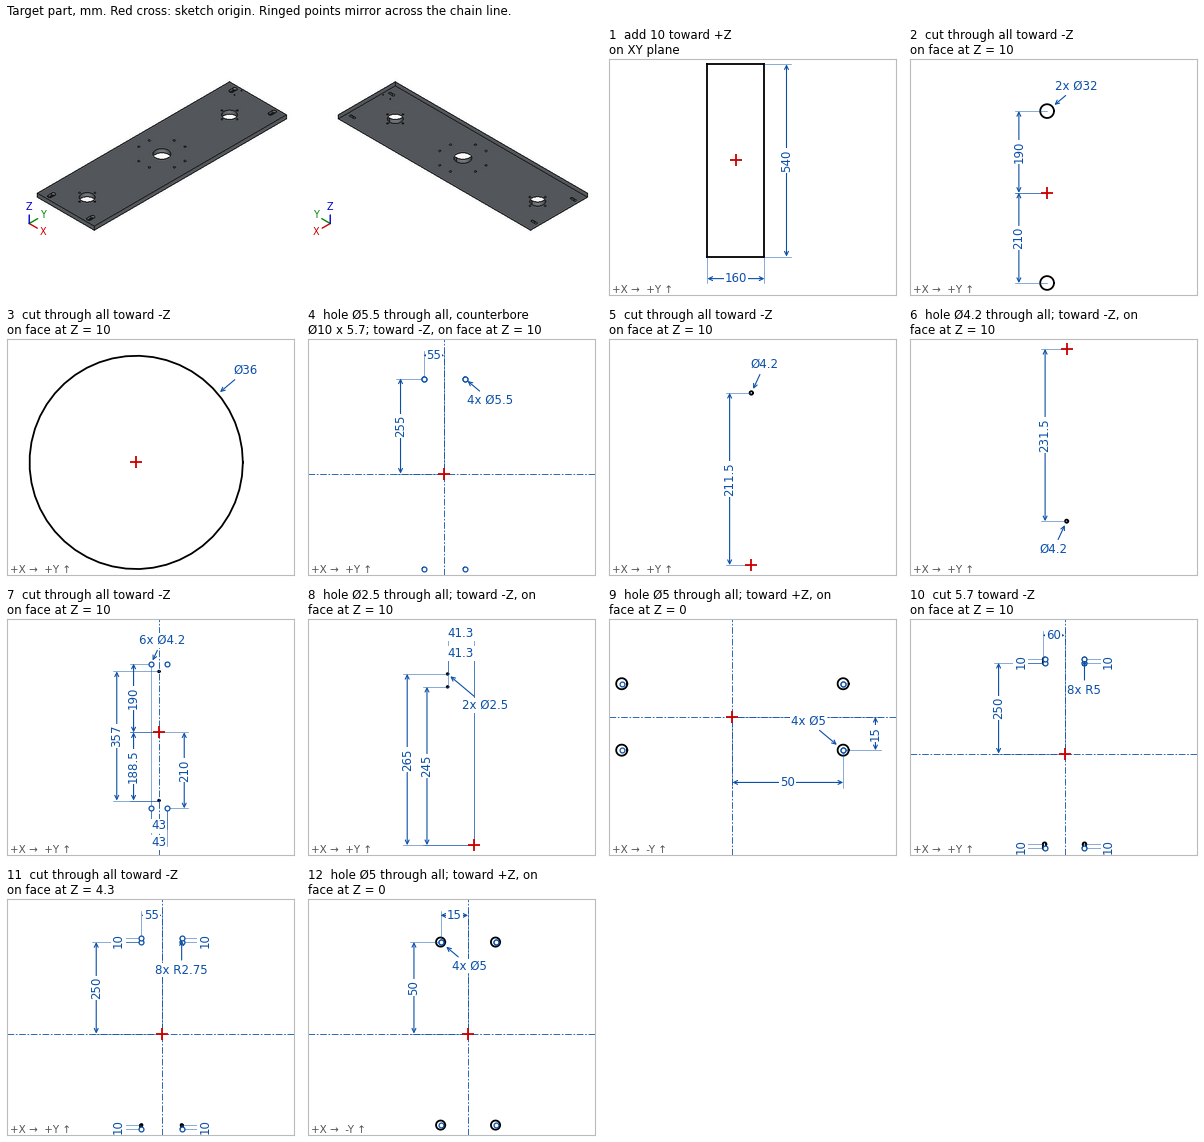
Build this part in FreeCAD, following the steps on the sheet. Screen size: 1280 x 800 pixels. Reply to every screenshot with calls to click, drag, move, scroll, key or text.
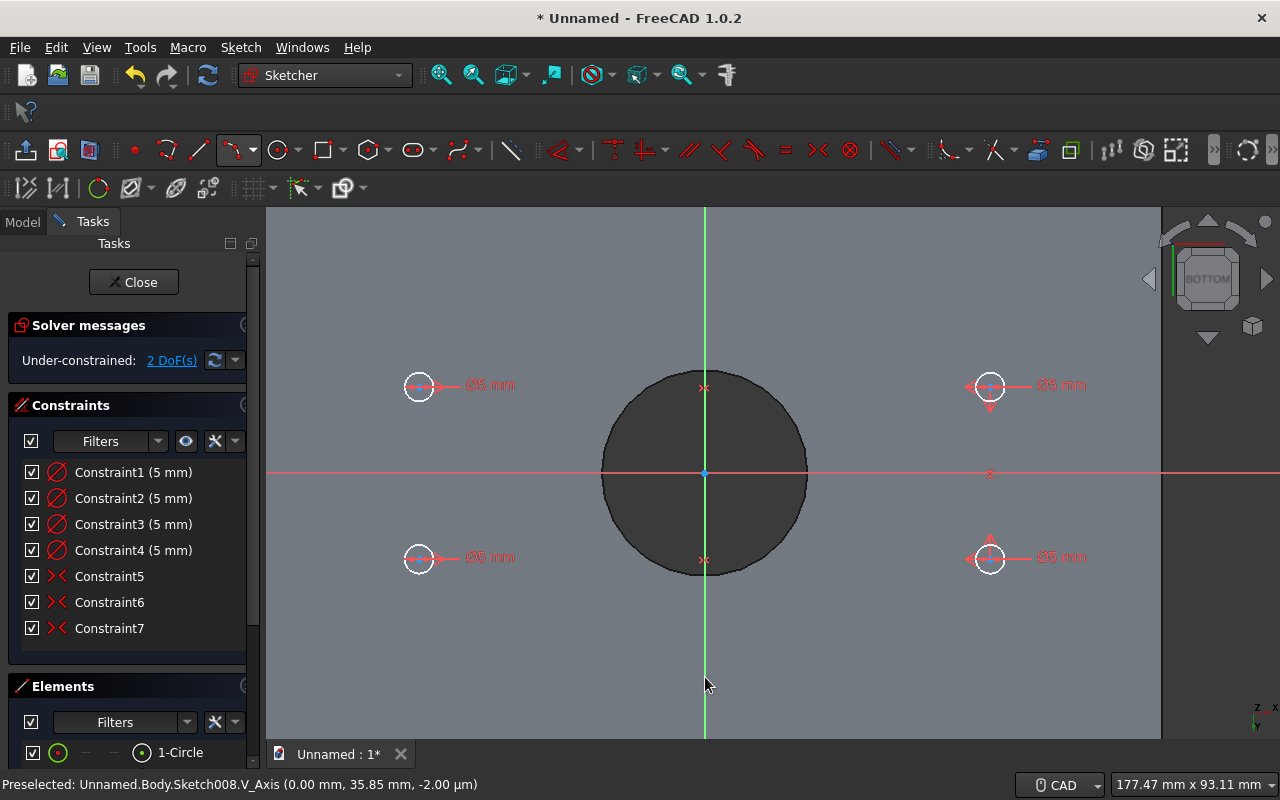
click(990, 559)
click(847, 593)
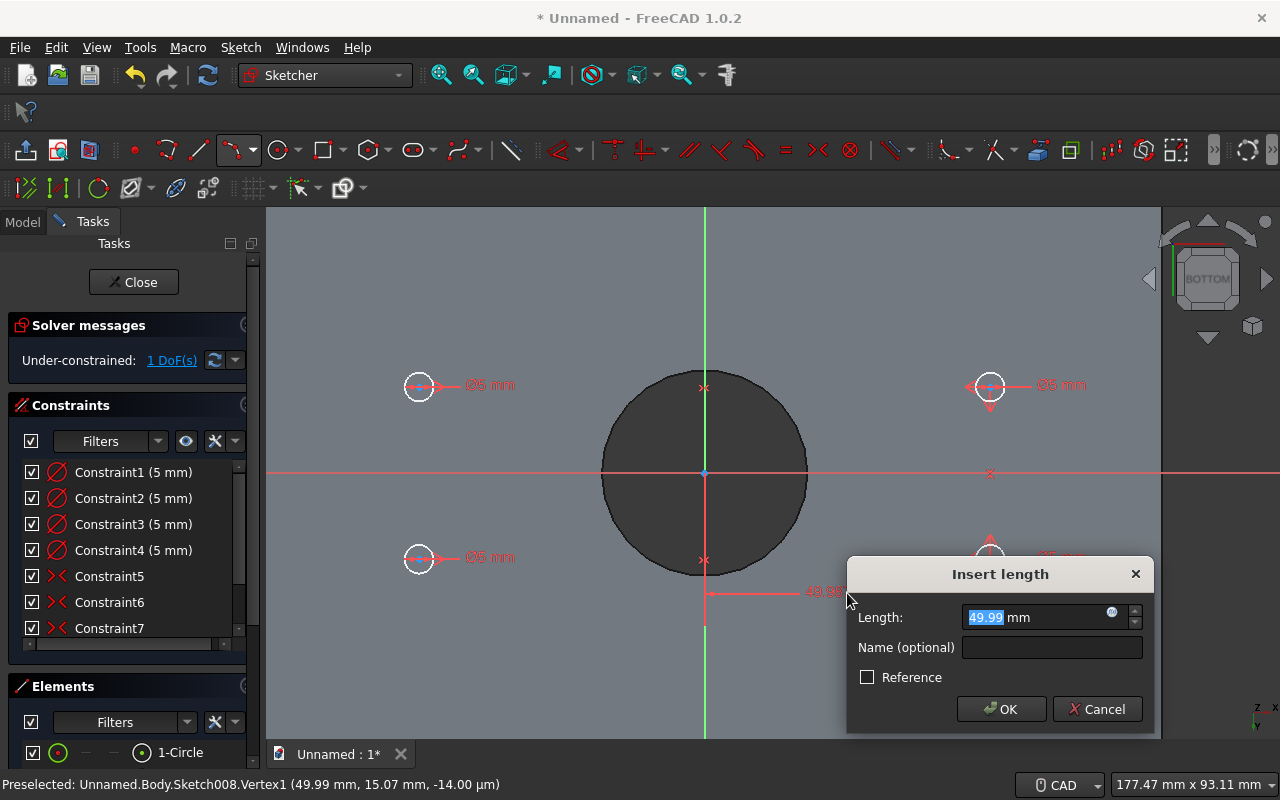
text(50)
key(Return)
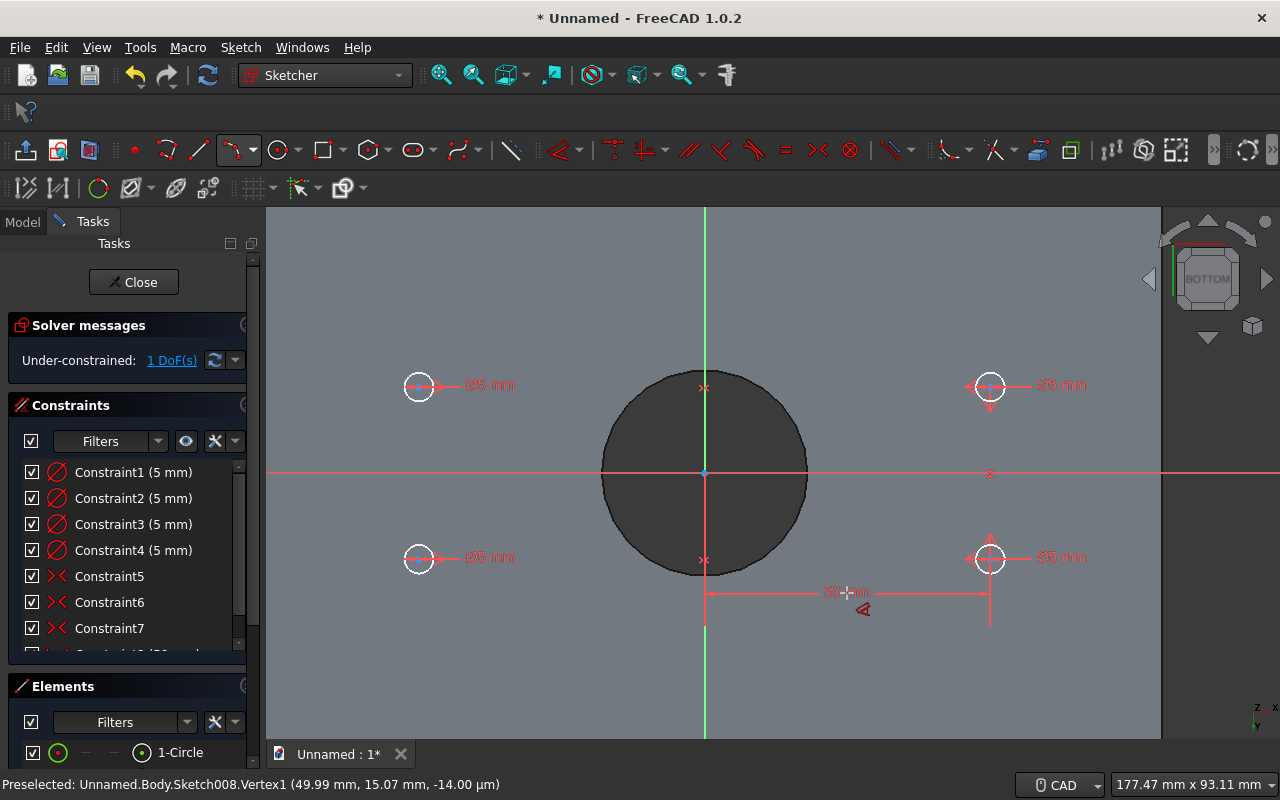
click(990, 559)
click(1024, 516)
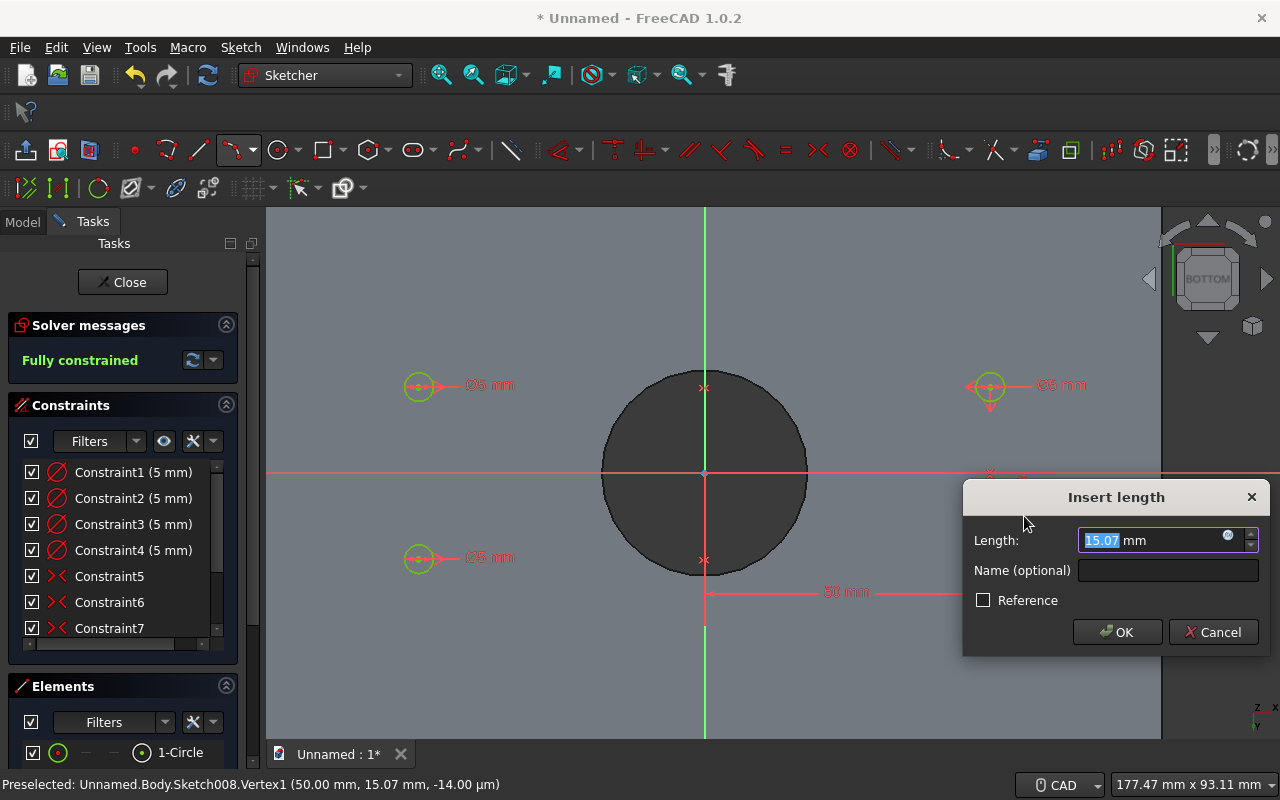
text(15)
key(Return)
key(Escape)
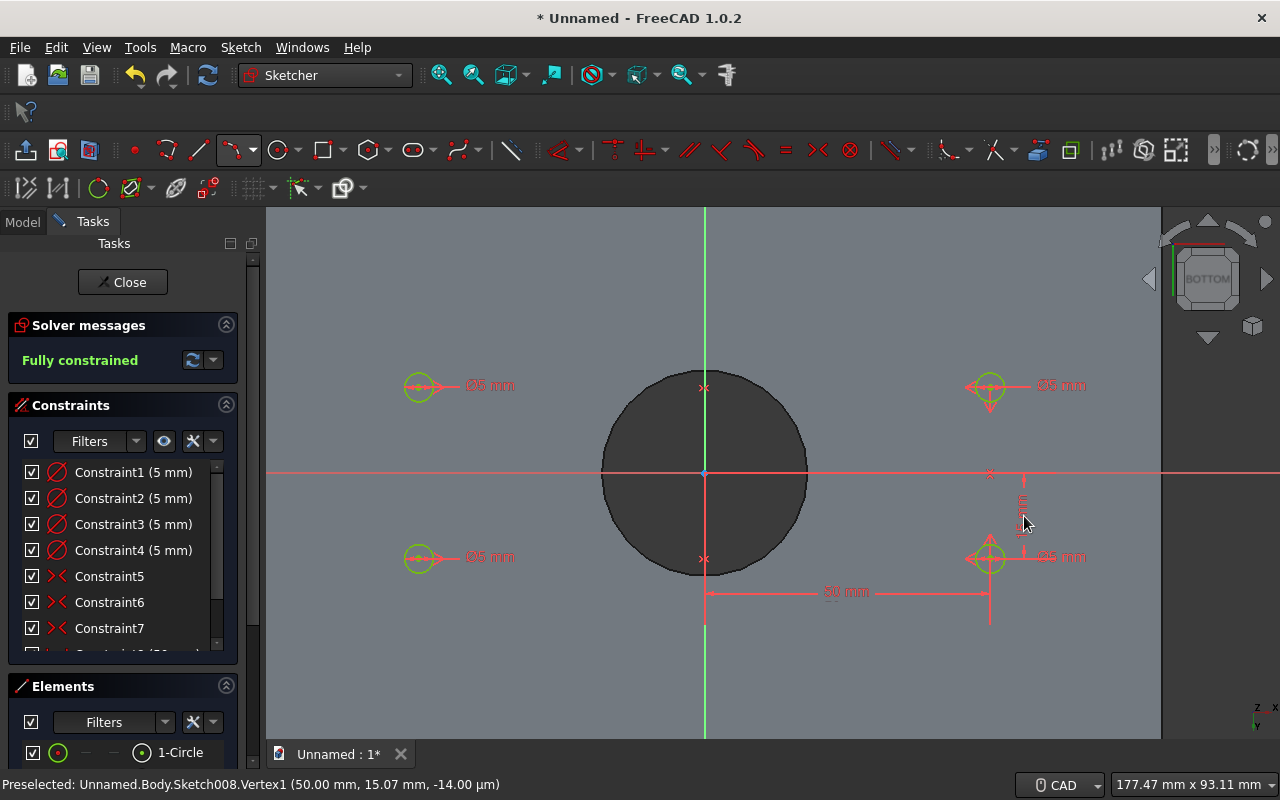
click(123, 282)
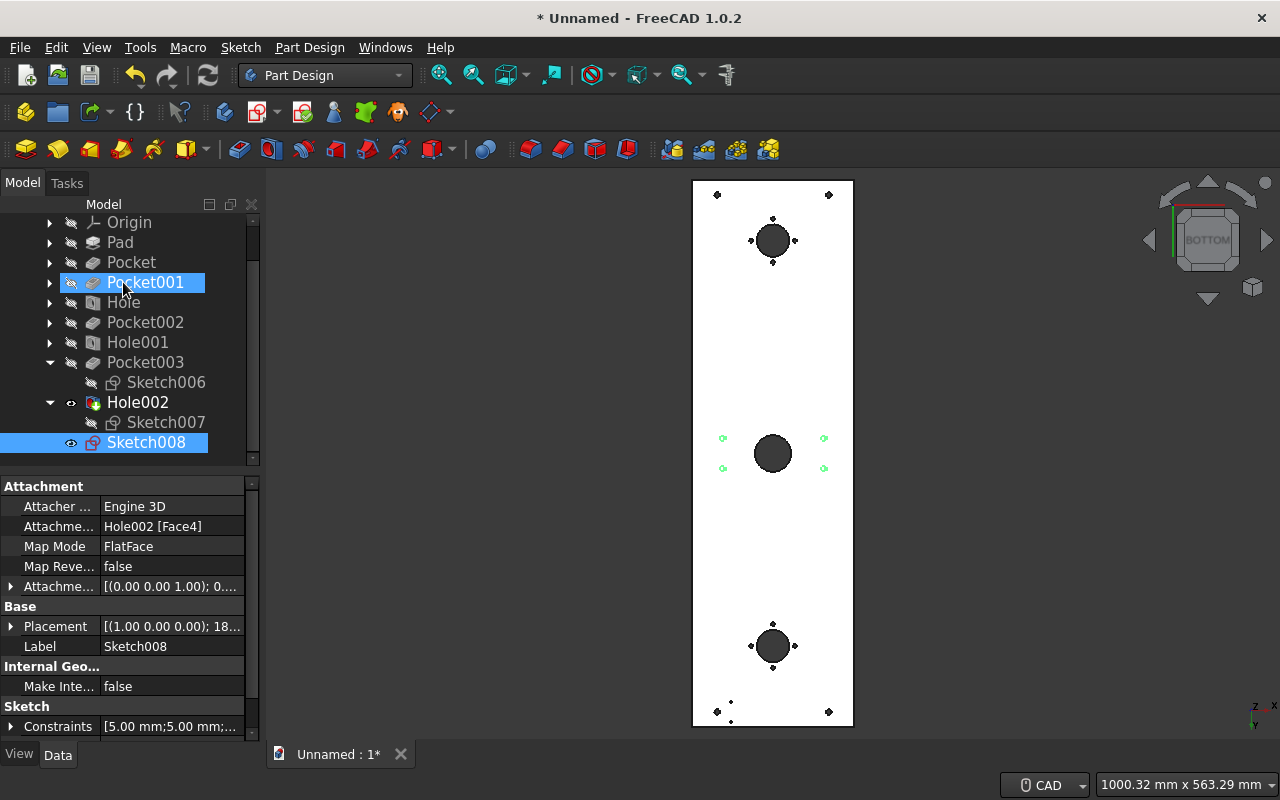
click(272, 150)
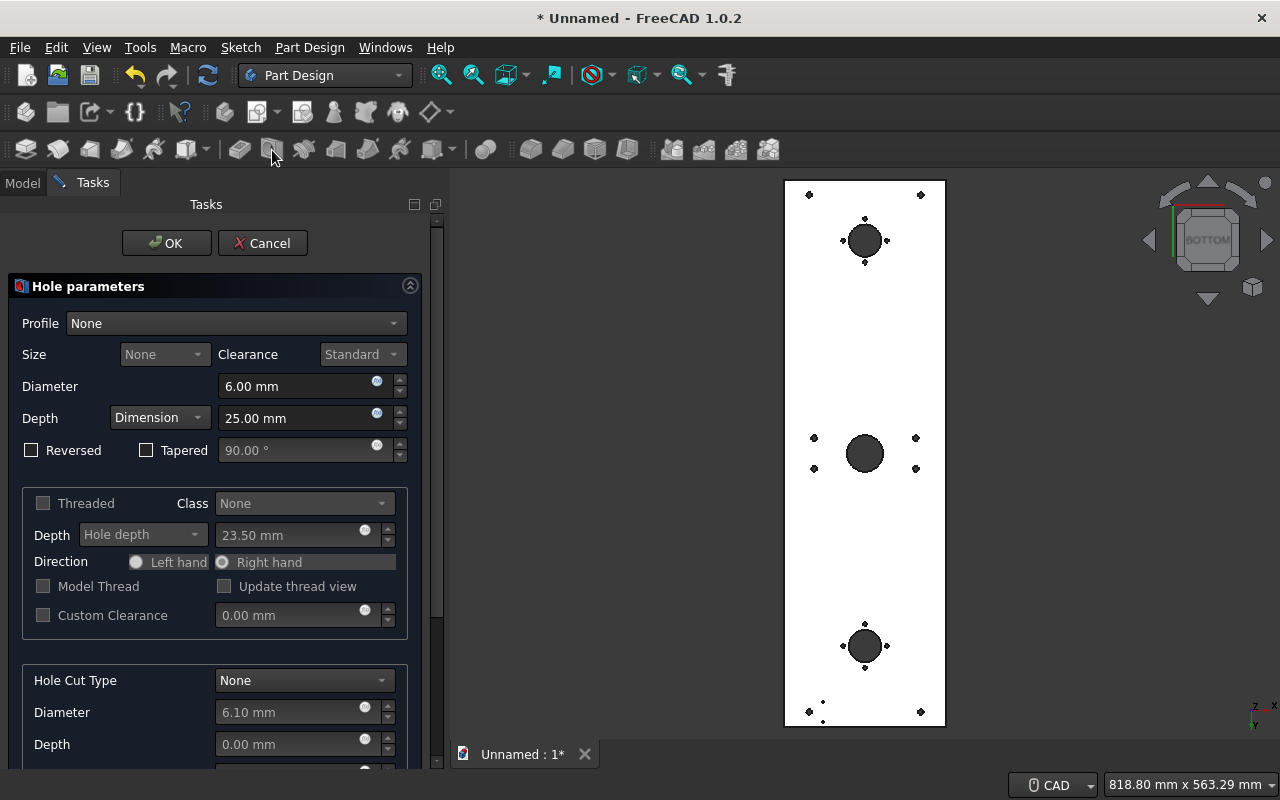
triple_click(305, 386)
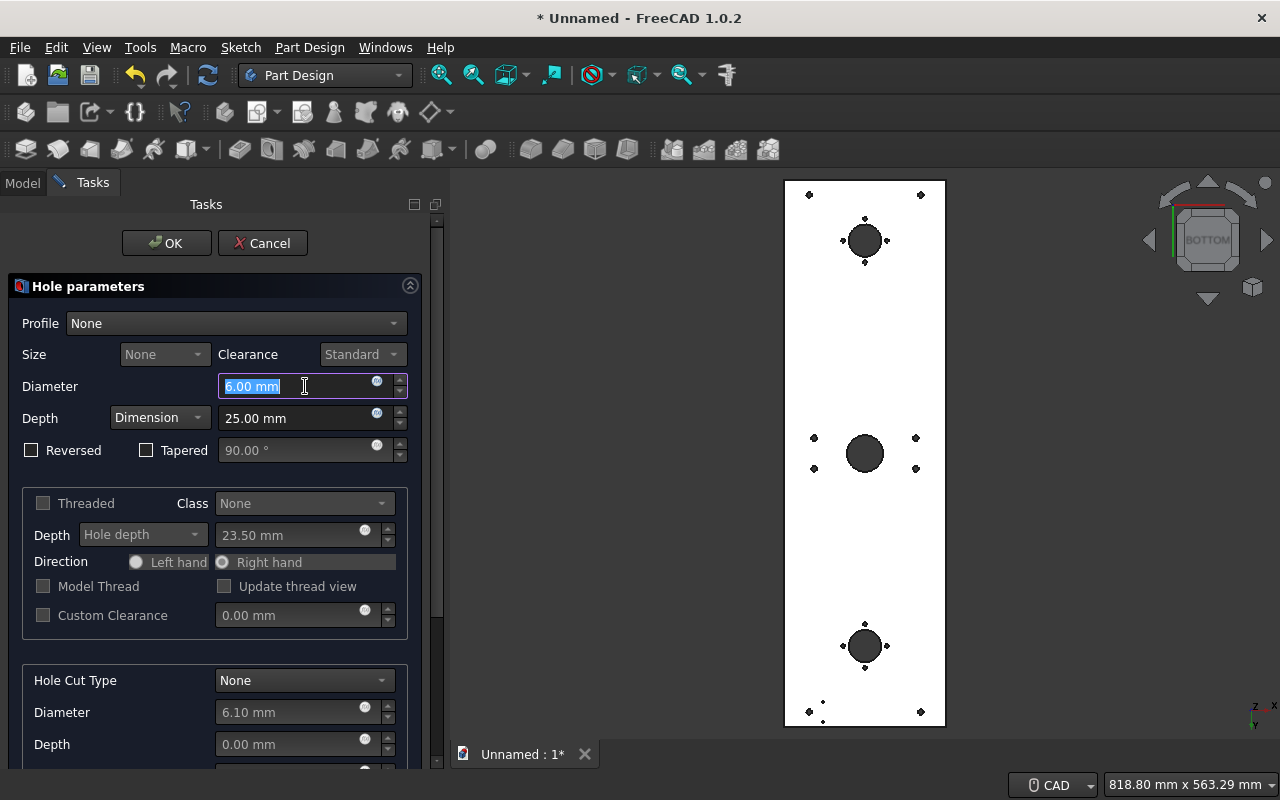
text(5)
key(Tab)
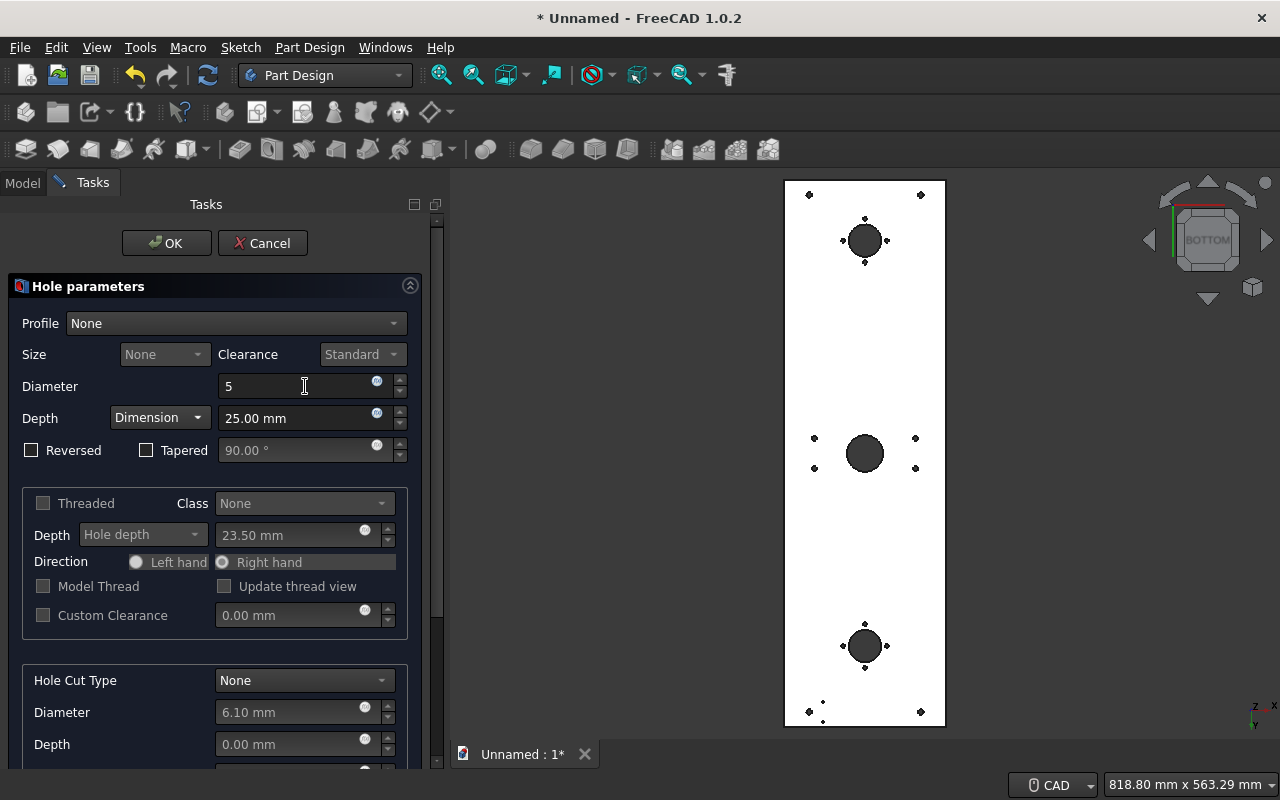
click(161, 418)